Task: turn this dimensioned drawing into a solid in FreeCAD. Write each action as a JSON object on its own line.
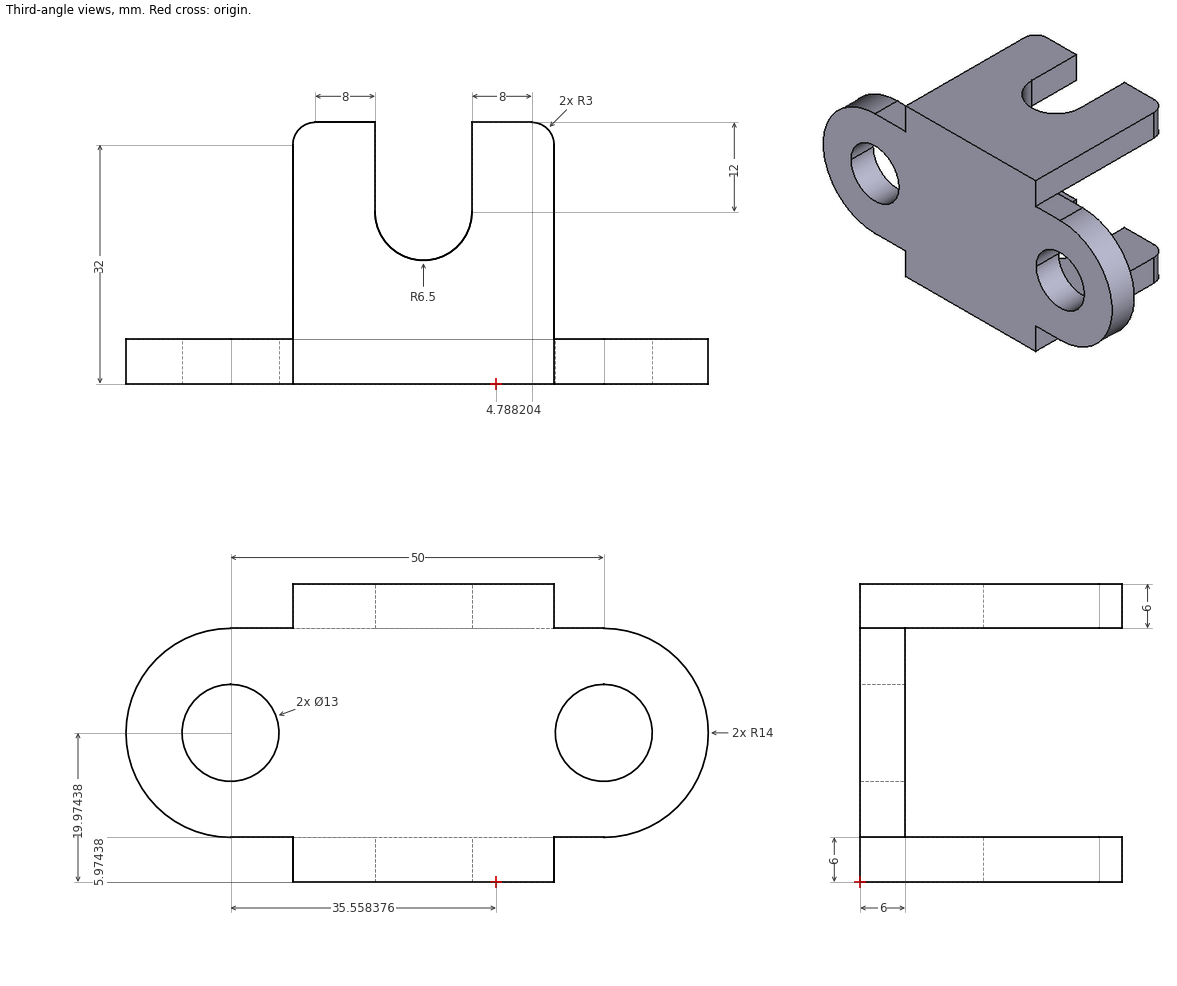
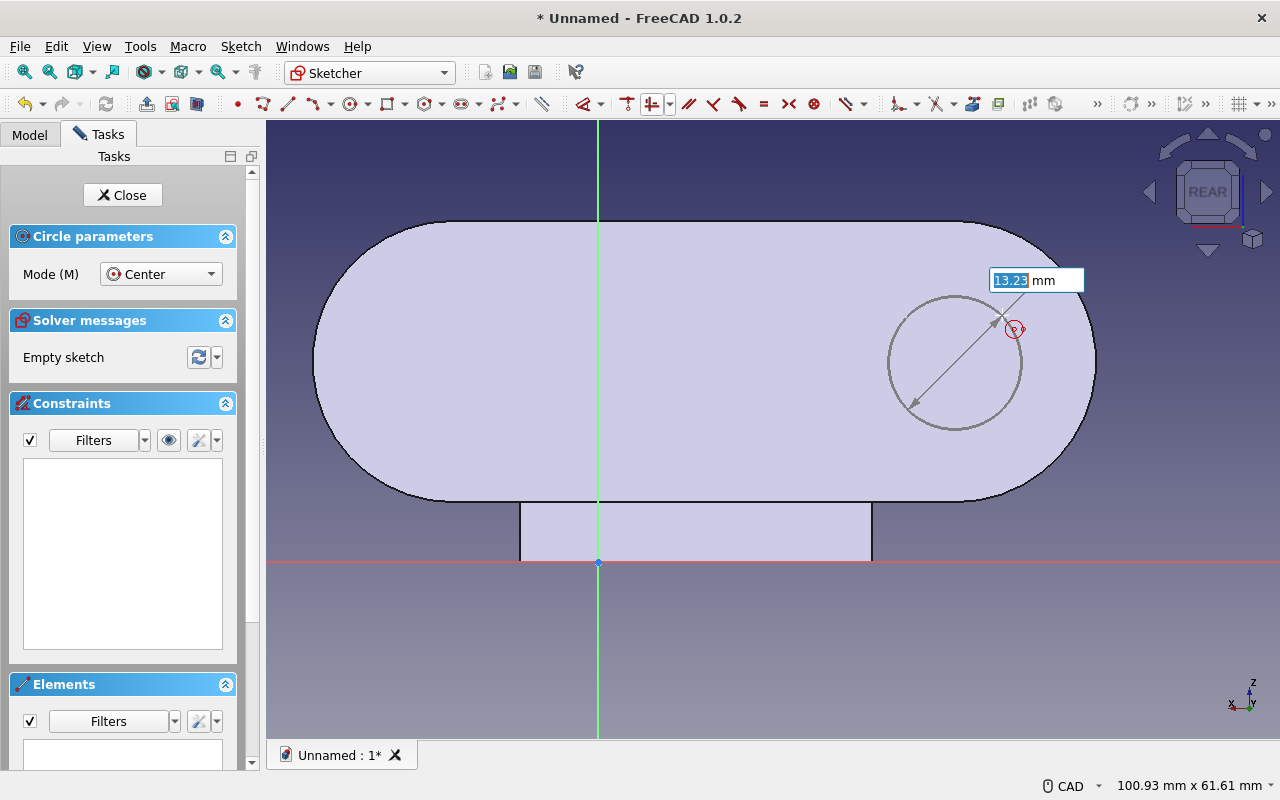
{"action": "type", "text": "13"}
{"action": "key", "text": "Return"}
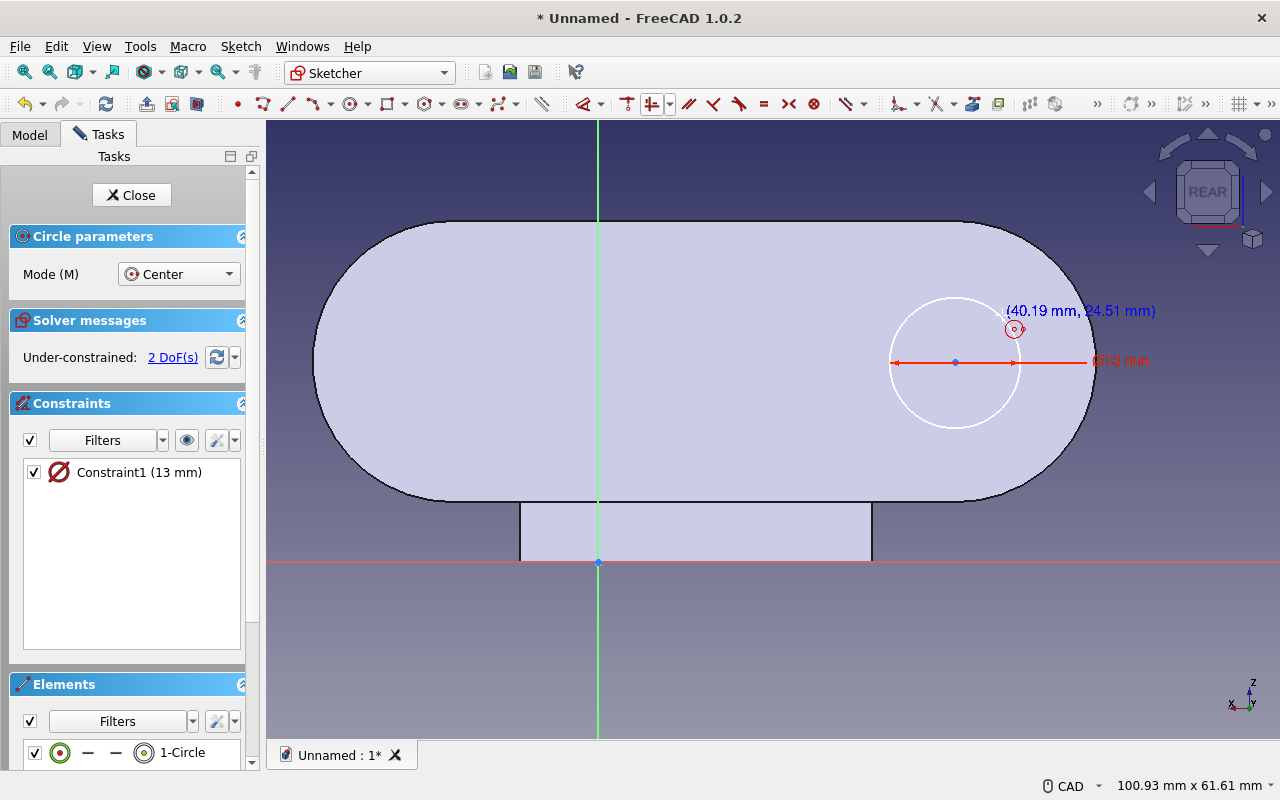
{"action": "left_click", "coordinate": [453, 362]}
{"action": "mouse_move", "coordinate": [499, 315]}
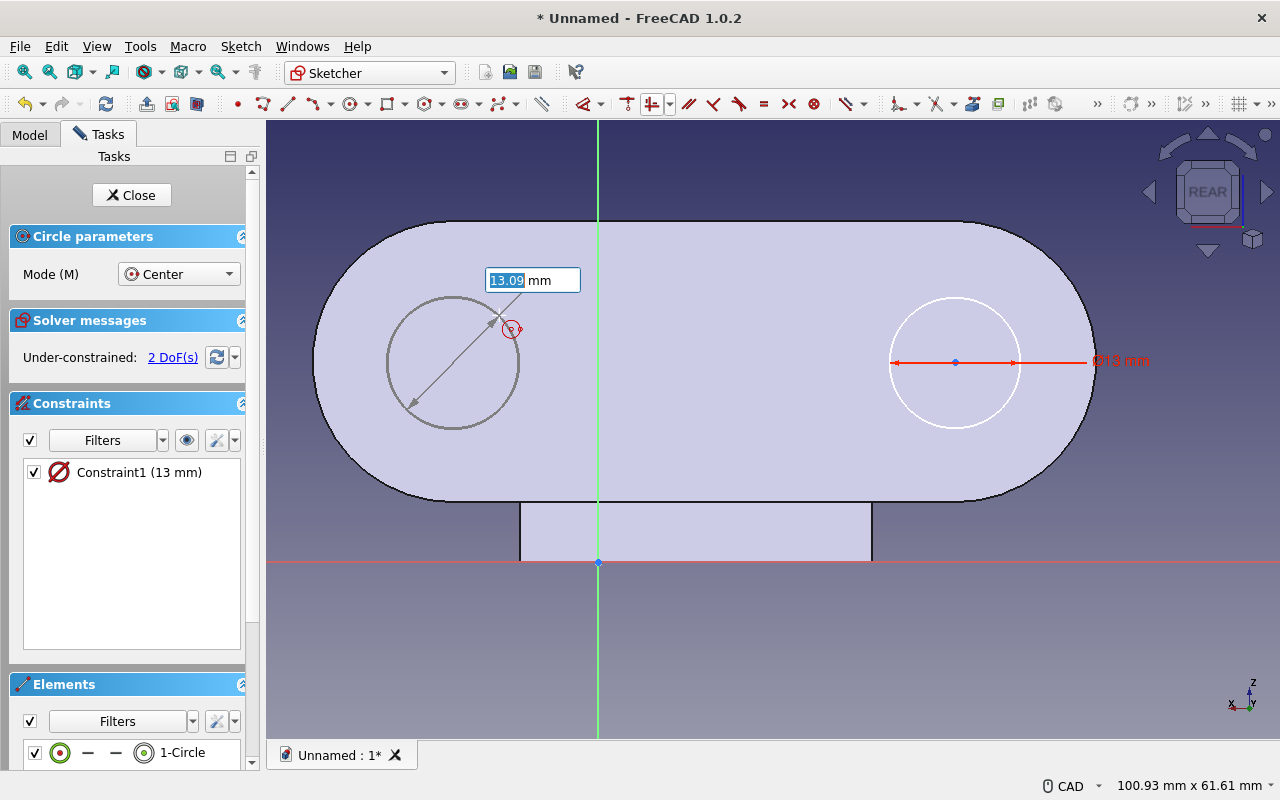
{"action": "type", "text": "13"}
{"action": "key", "text": "Return"}
{"action": "key", "text": "Escape"}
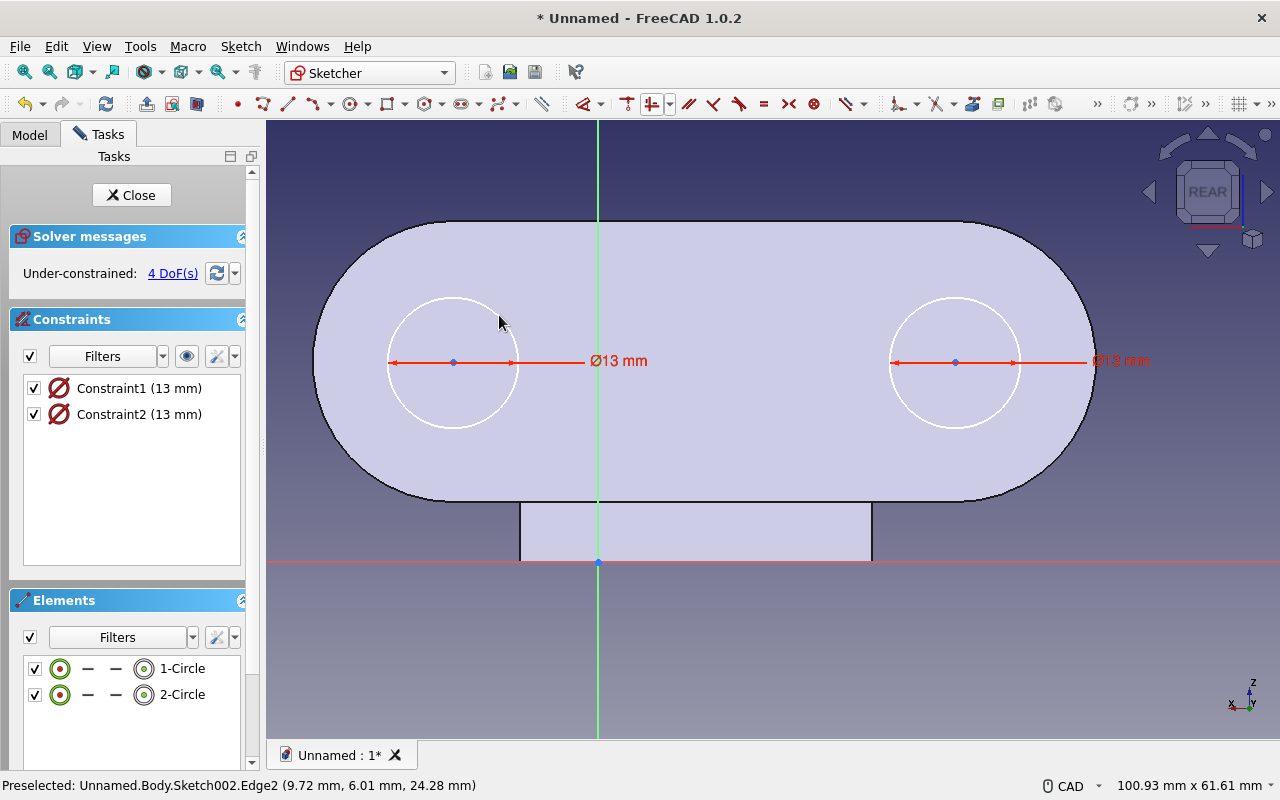
{"action": "left_click", "coordinate": [955, 363]}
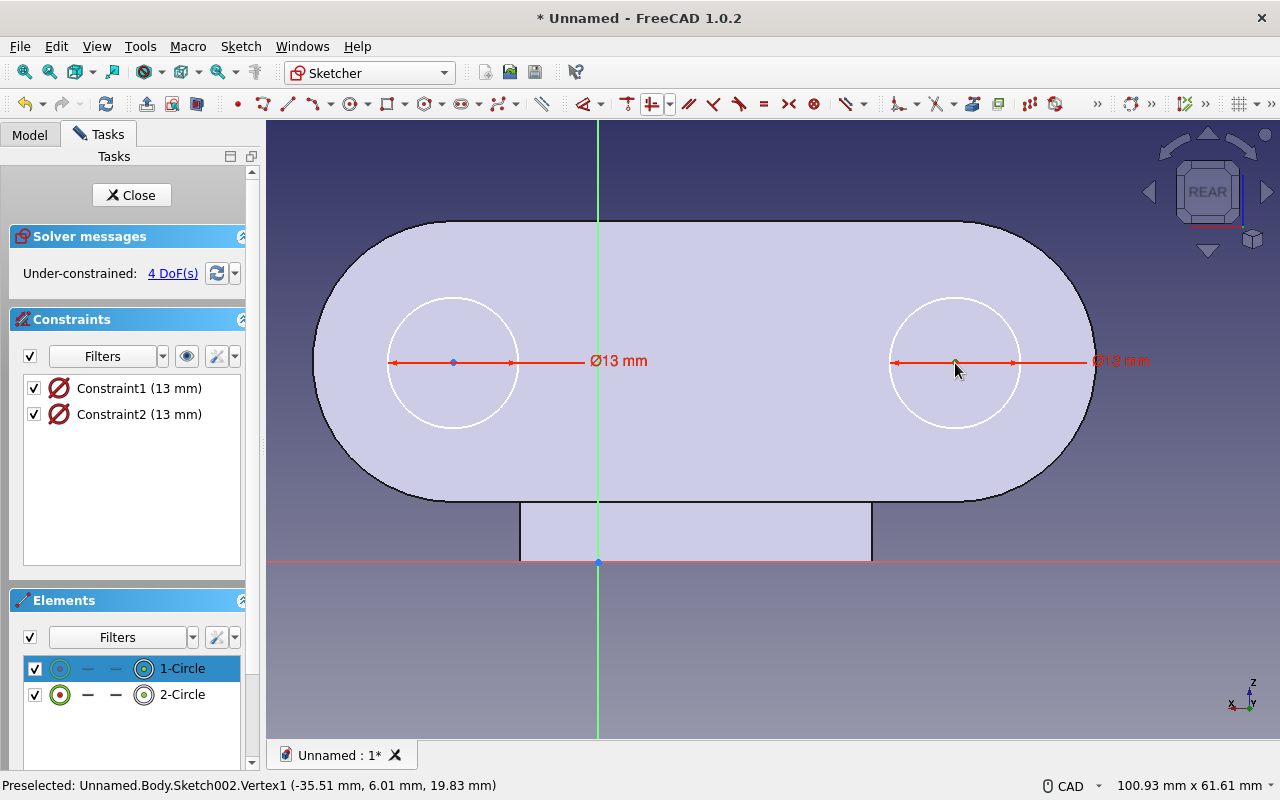
{"action": "left_click", "coordinate": [453, 363]}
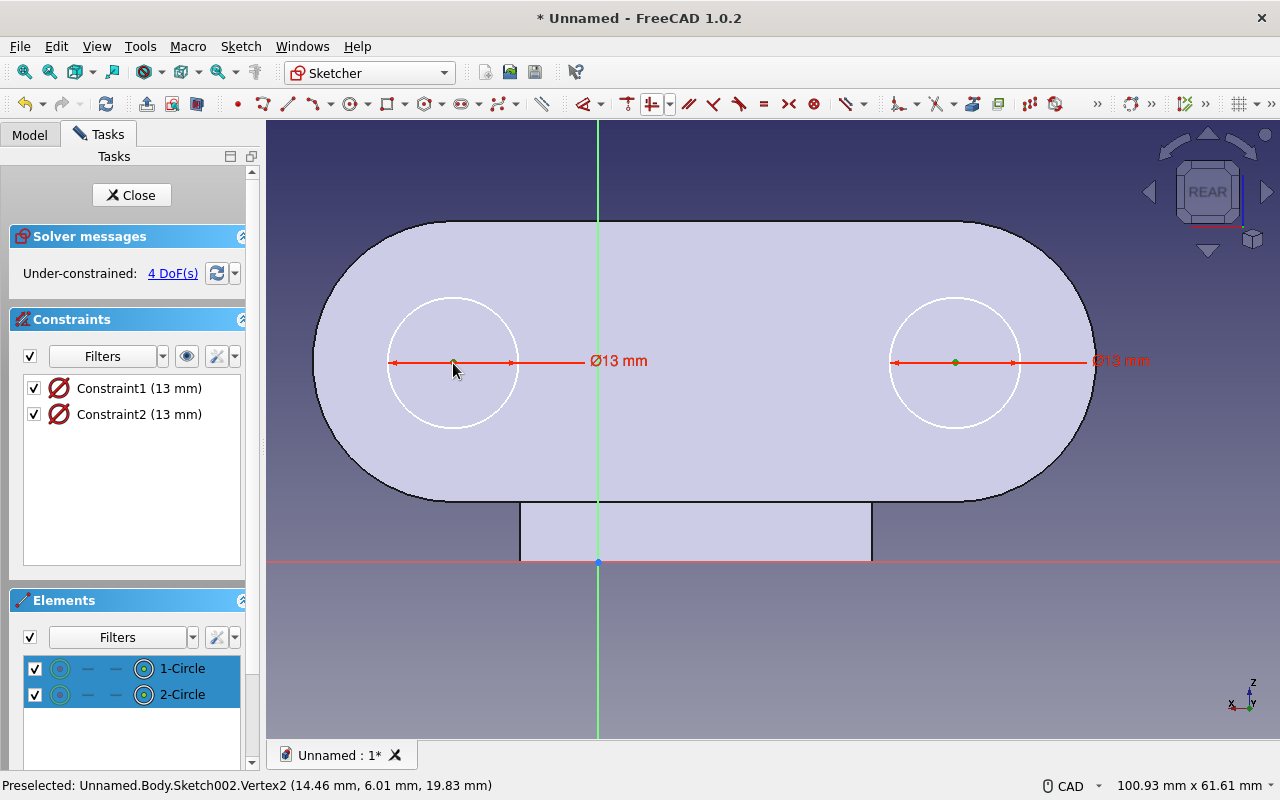
{"action": "left_click", "coordinate": [670, 104]}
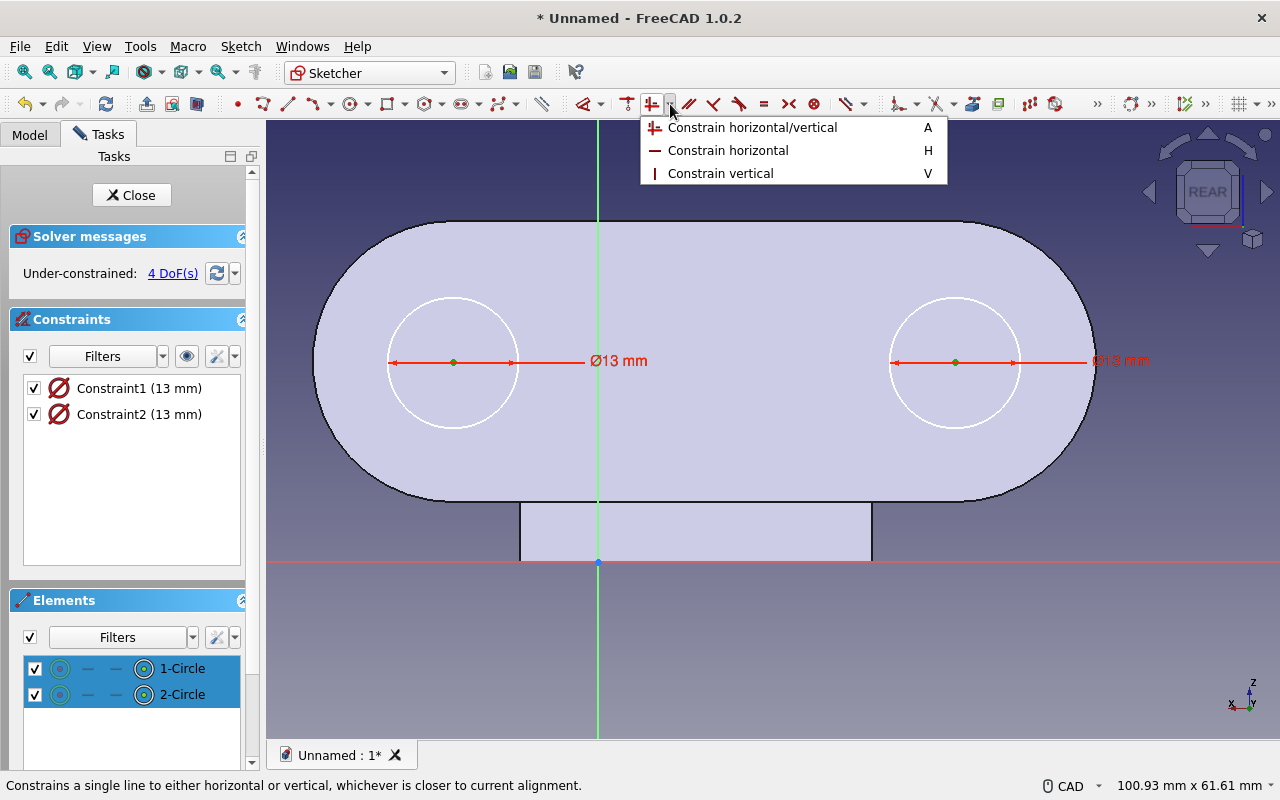
{"action": "left_click", "coordinate": [794, 150]}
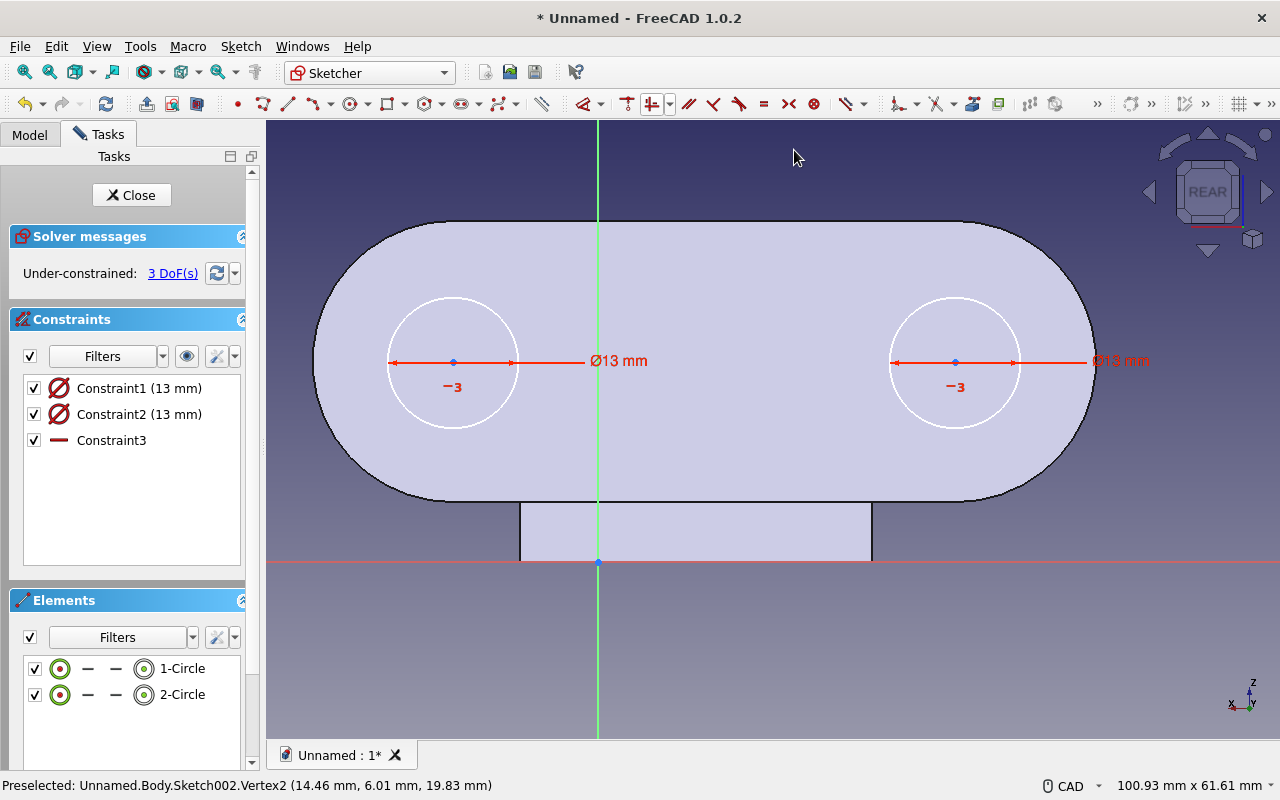
{"action": "left_click", "coordinate": [582, 104]}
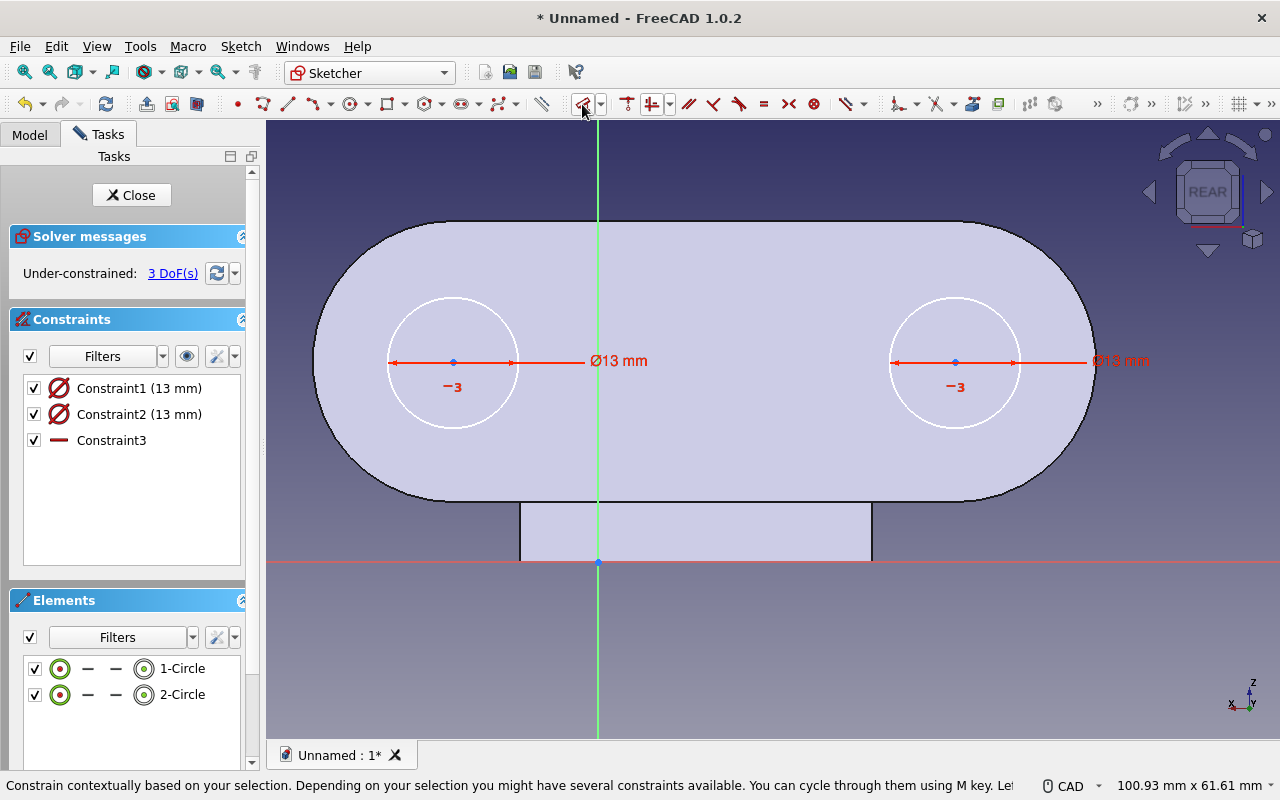
{"action": "left_click", "coordinate": [955, 363]}